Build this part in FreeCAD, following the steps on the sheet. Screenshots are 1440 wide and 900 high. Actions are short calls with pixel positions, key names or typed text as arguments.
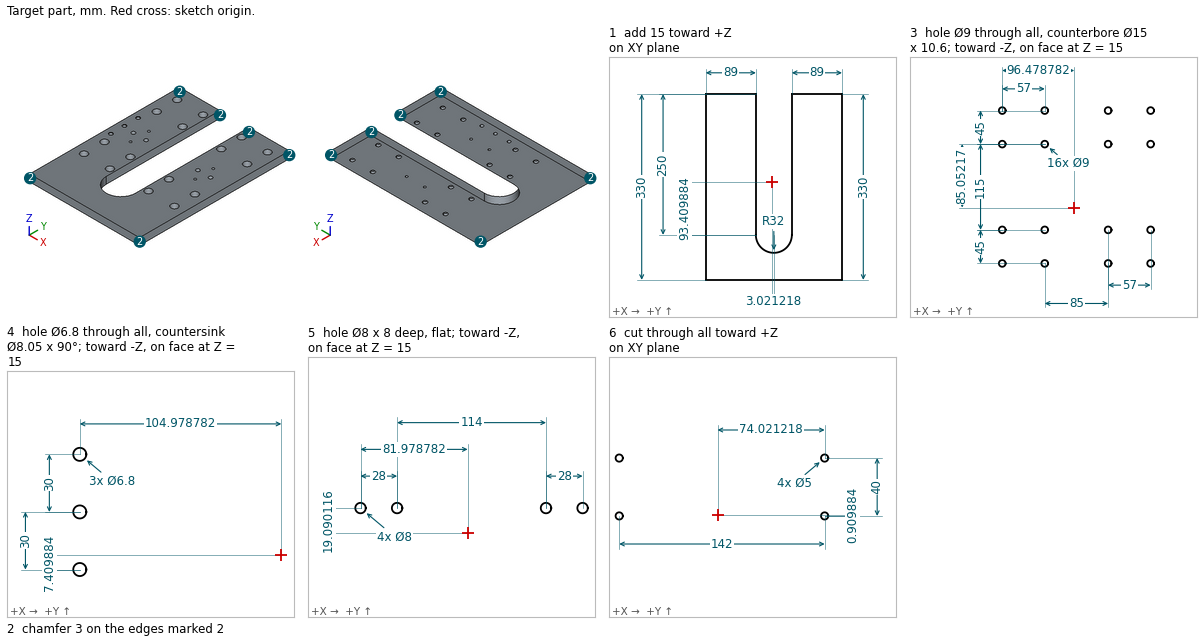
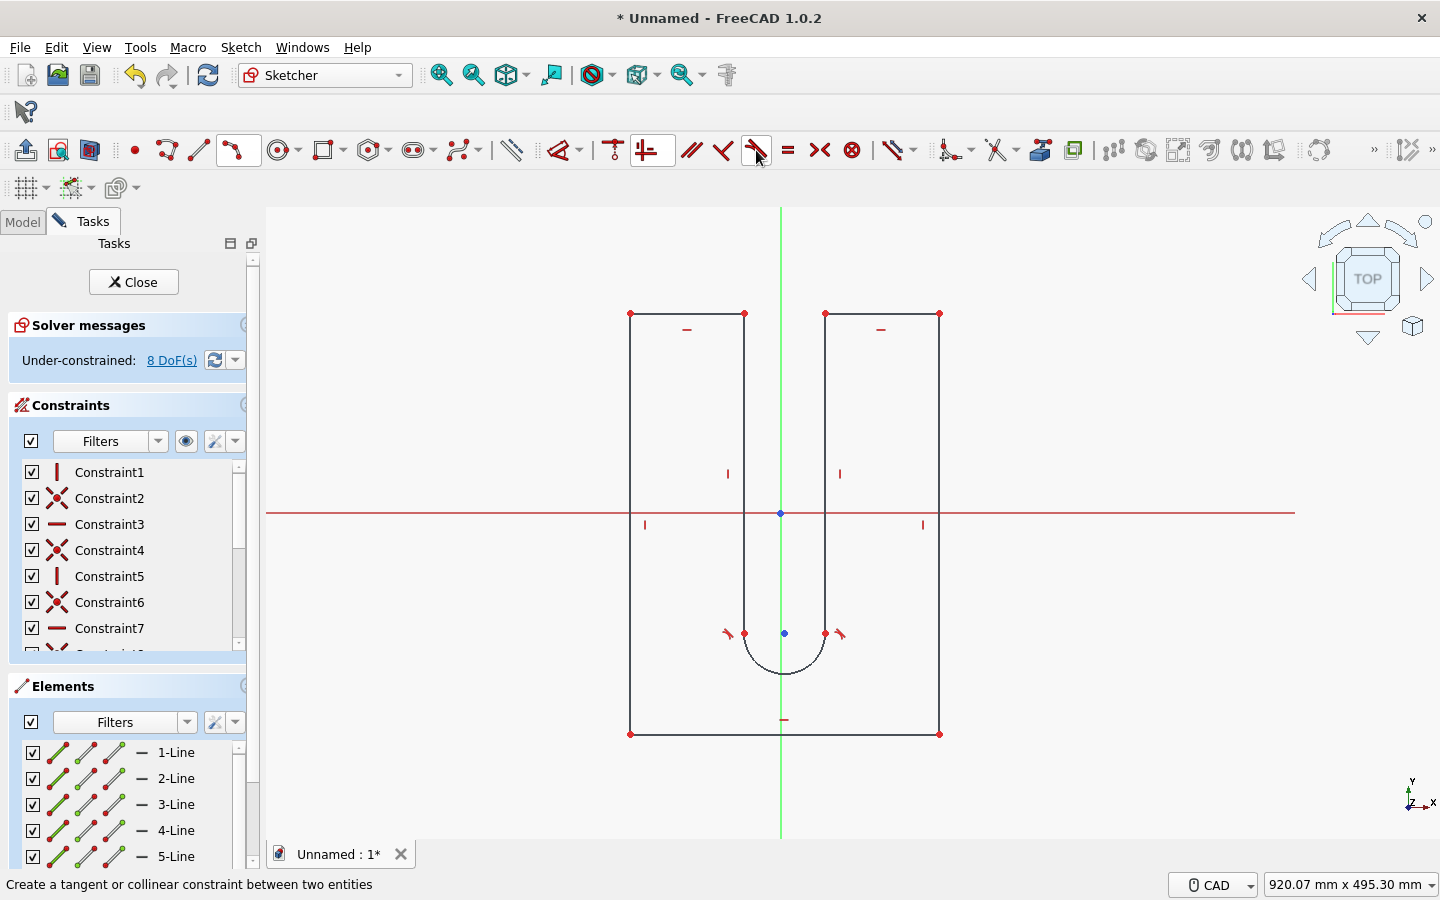
click(558, 150)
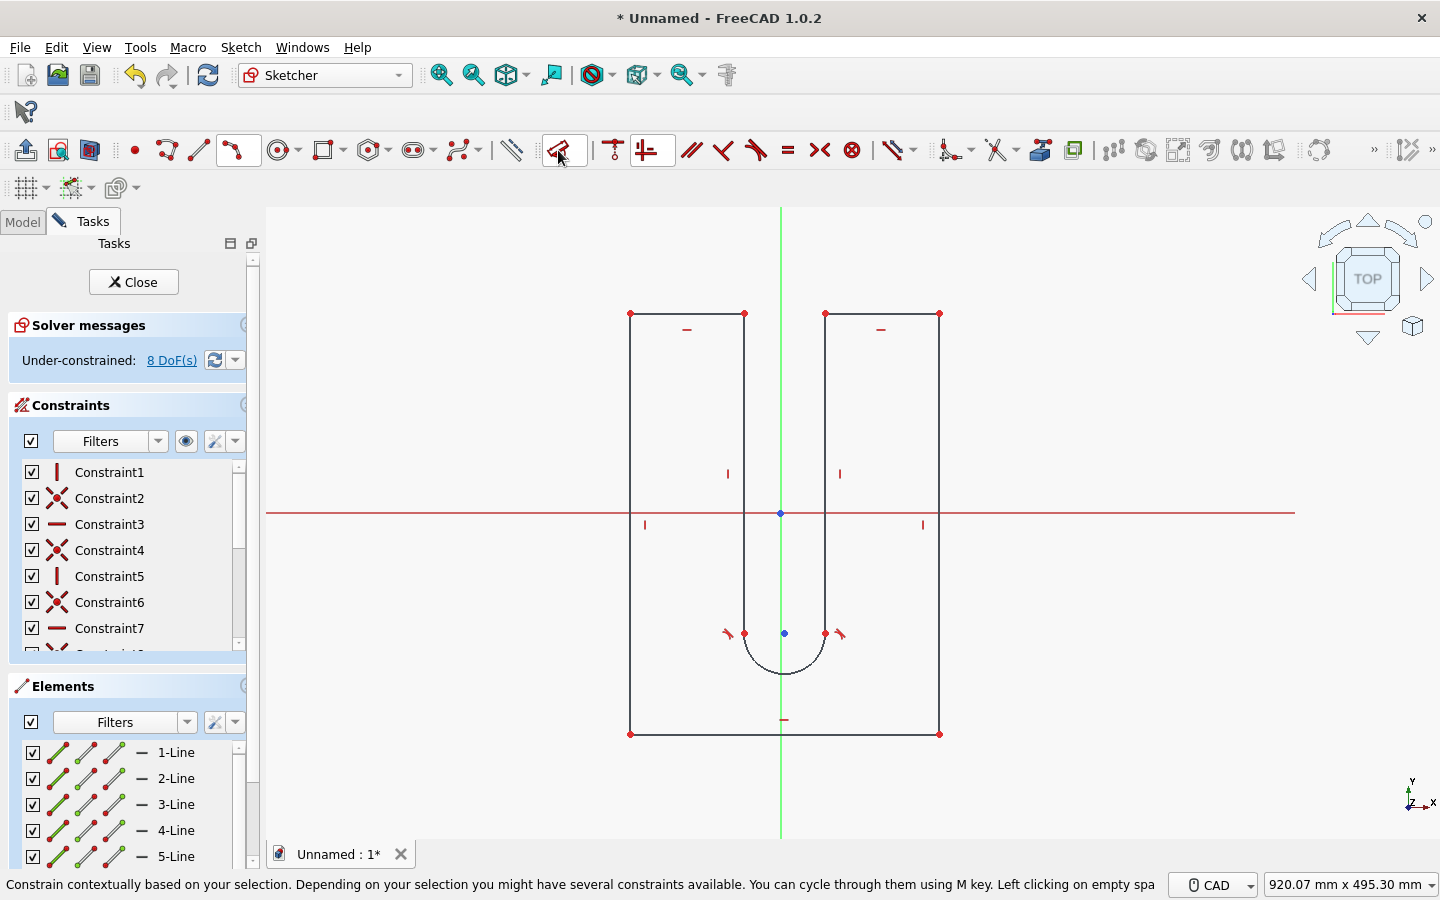
click(761, 666)
click(742, 692)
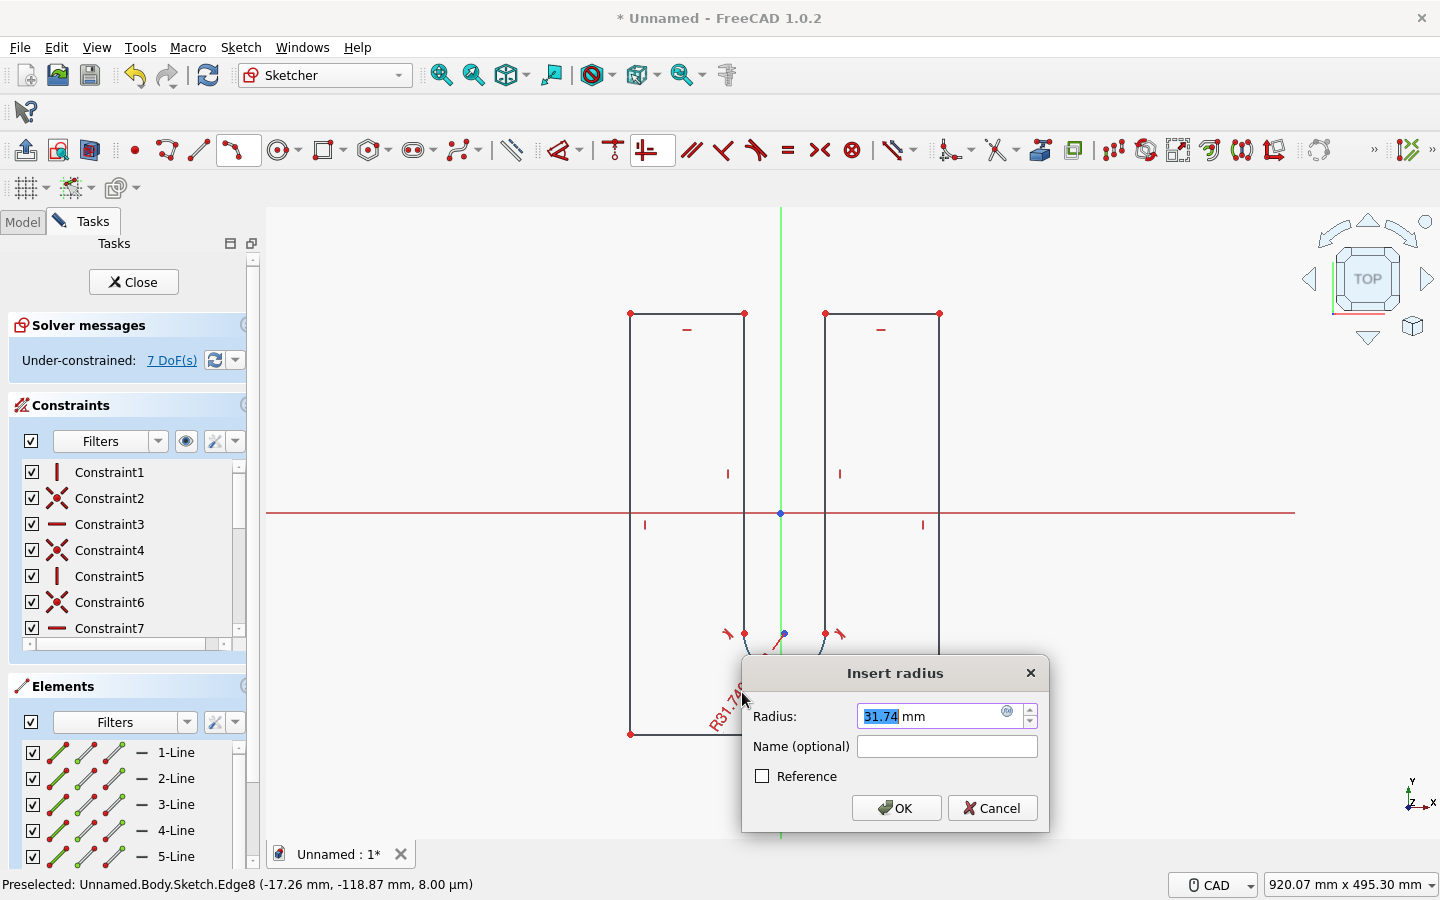
text(32)
key(Return)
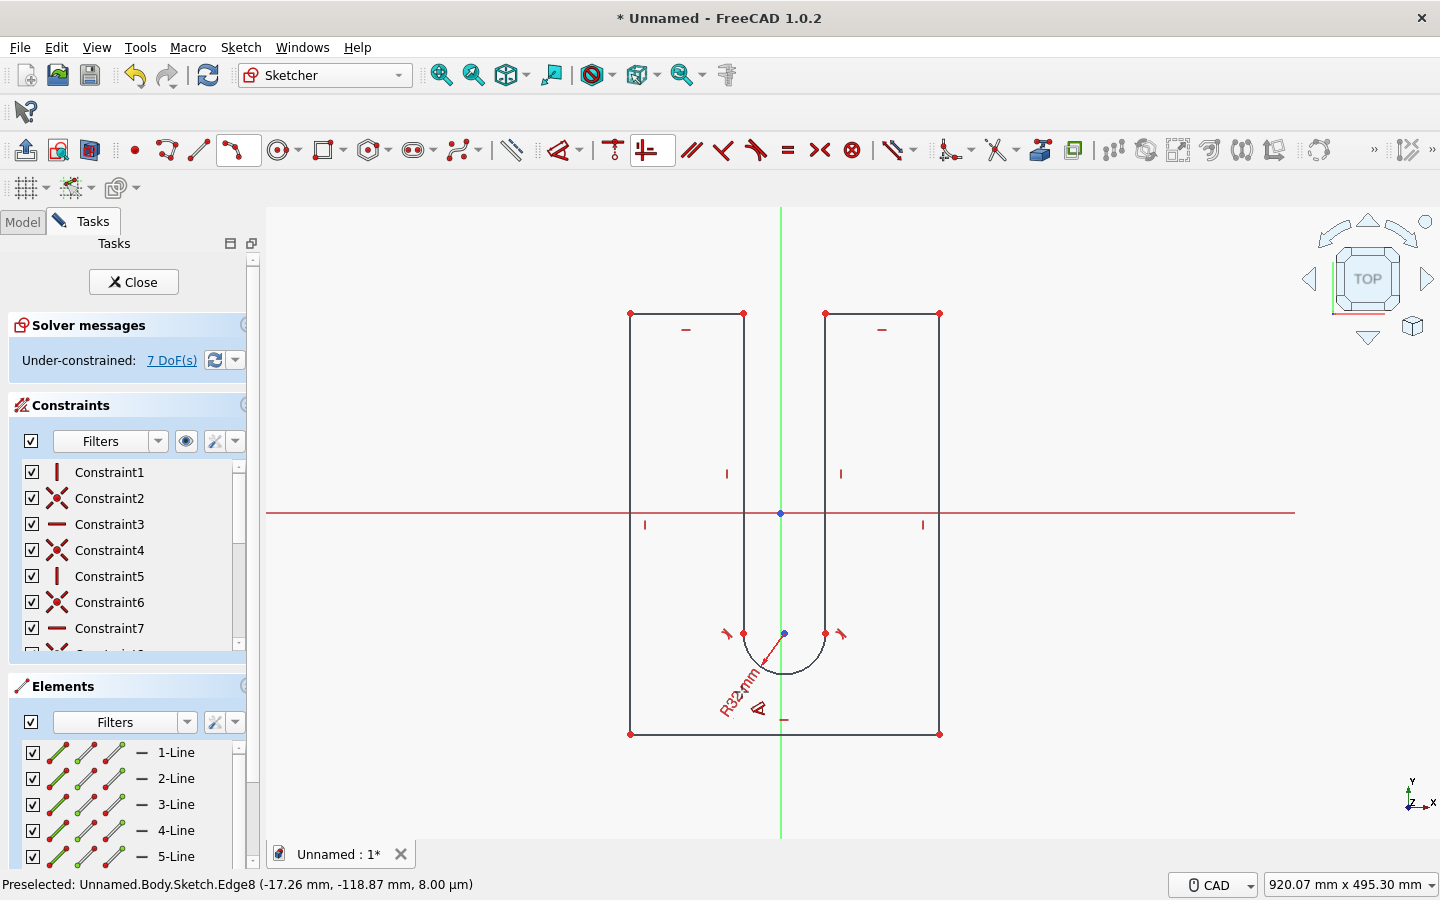
click(710, 314)
click(687, 280)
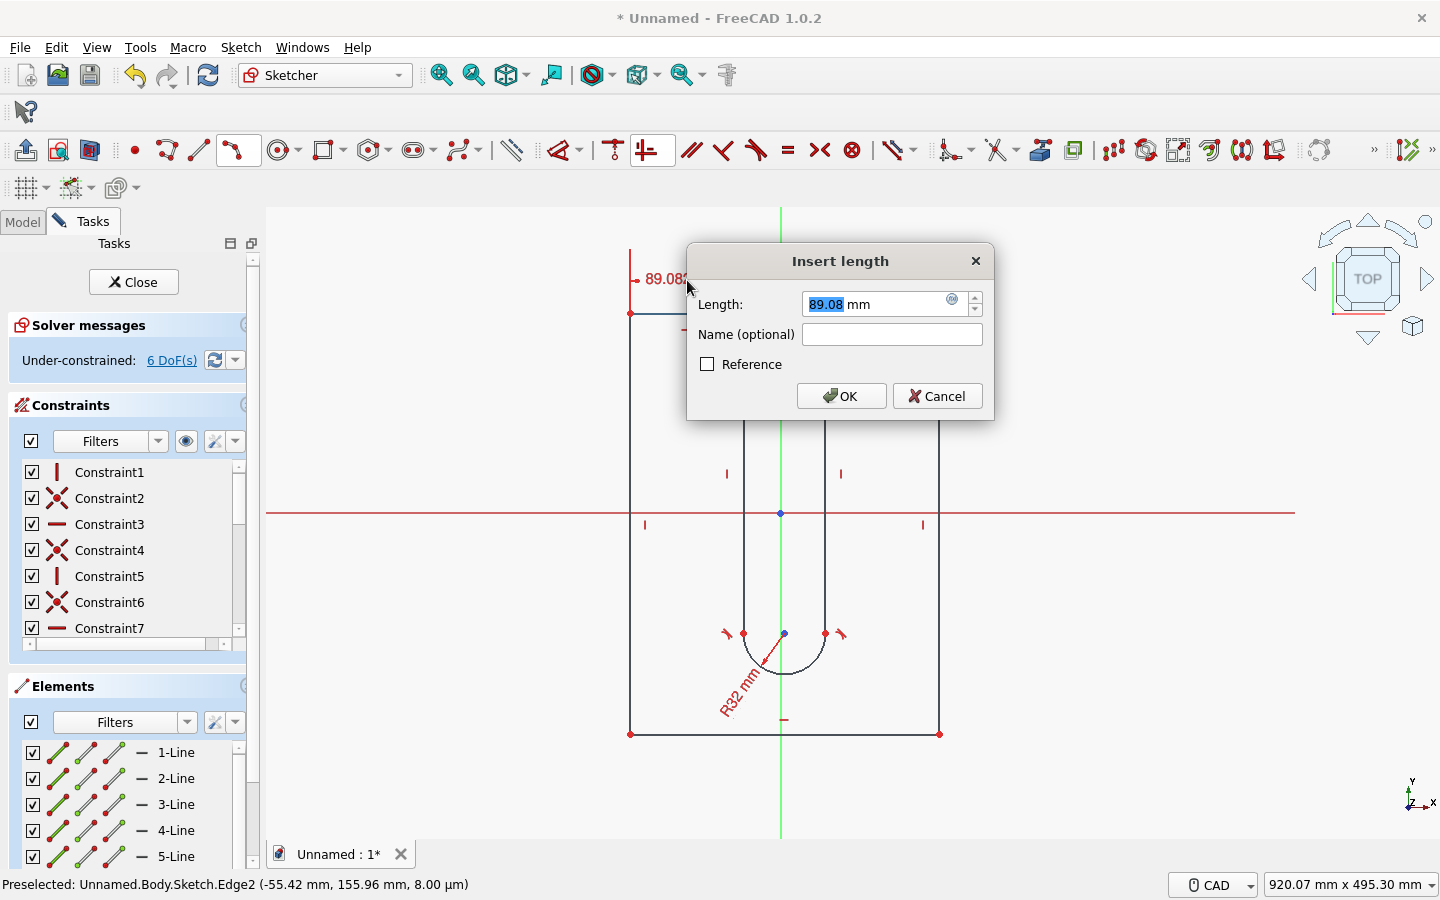
text(89)
key(Return)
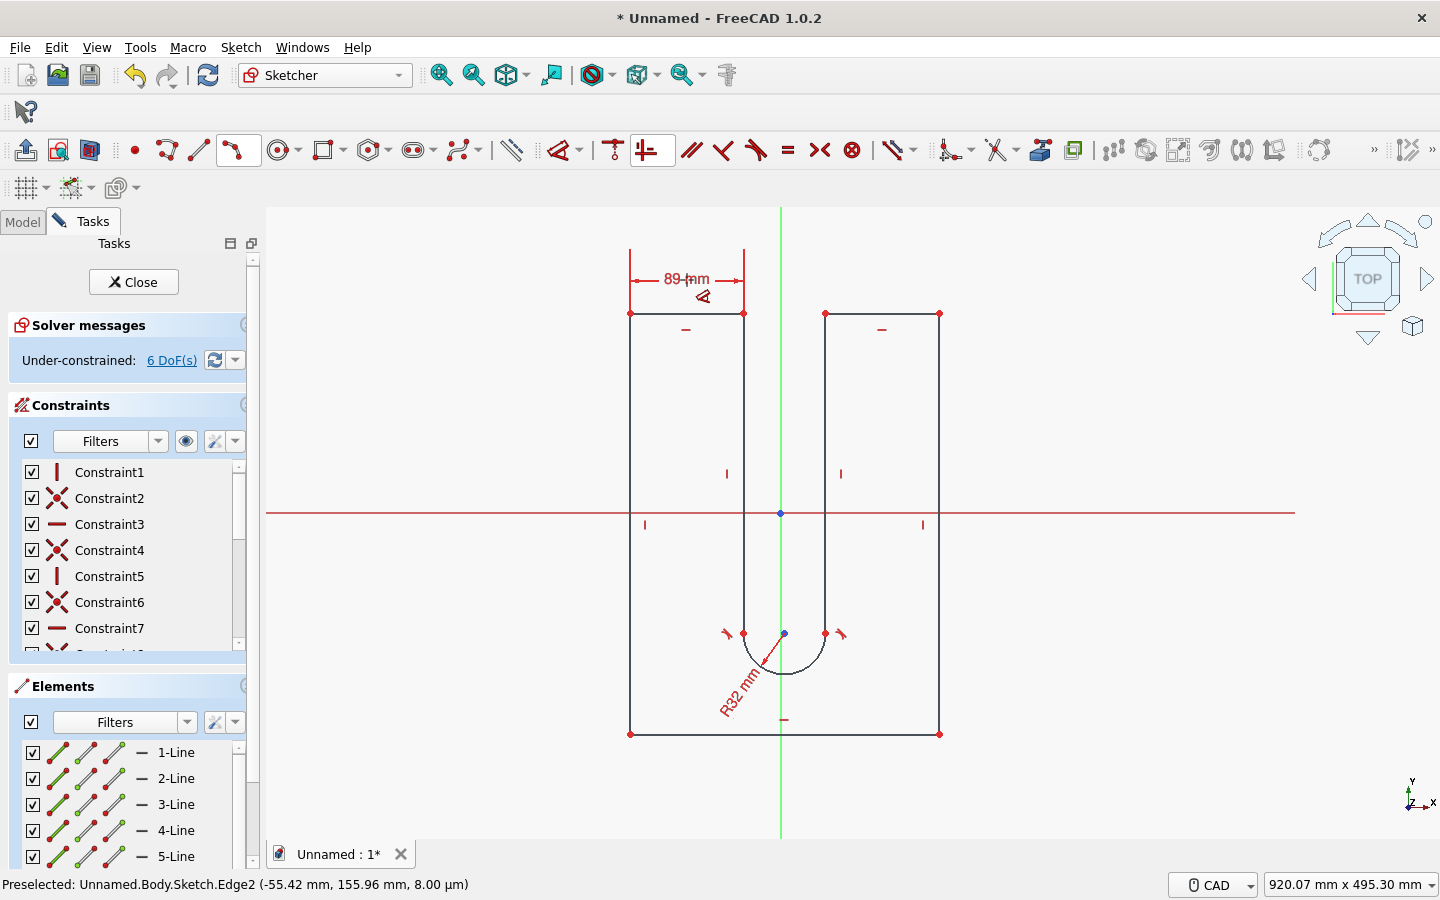
click(905, 314)
click(882, 280)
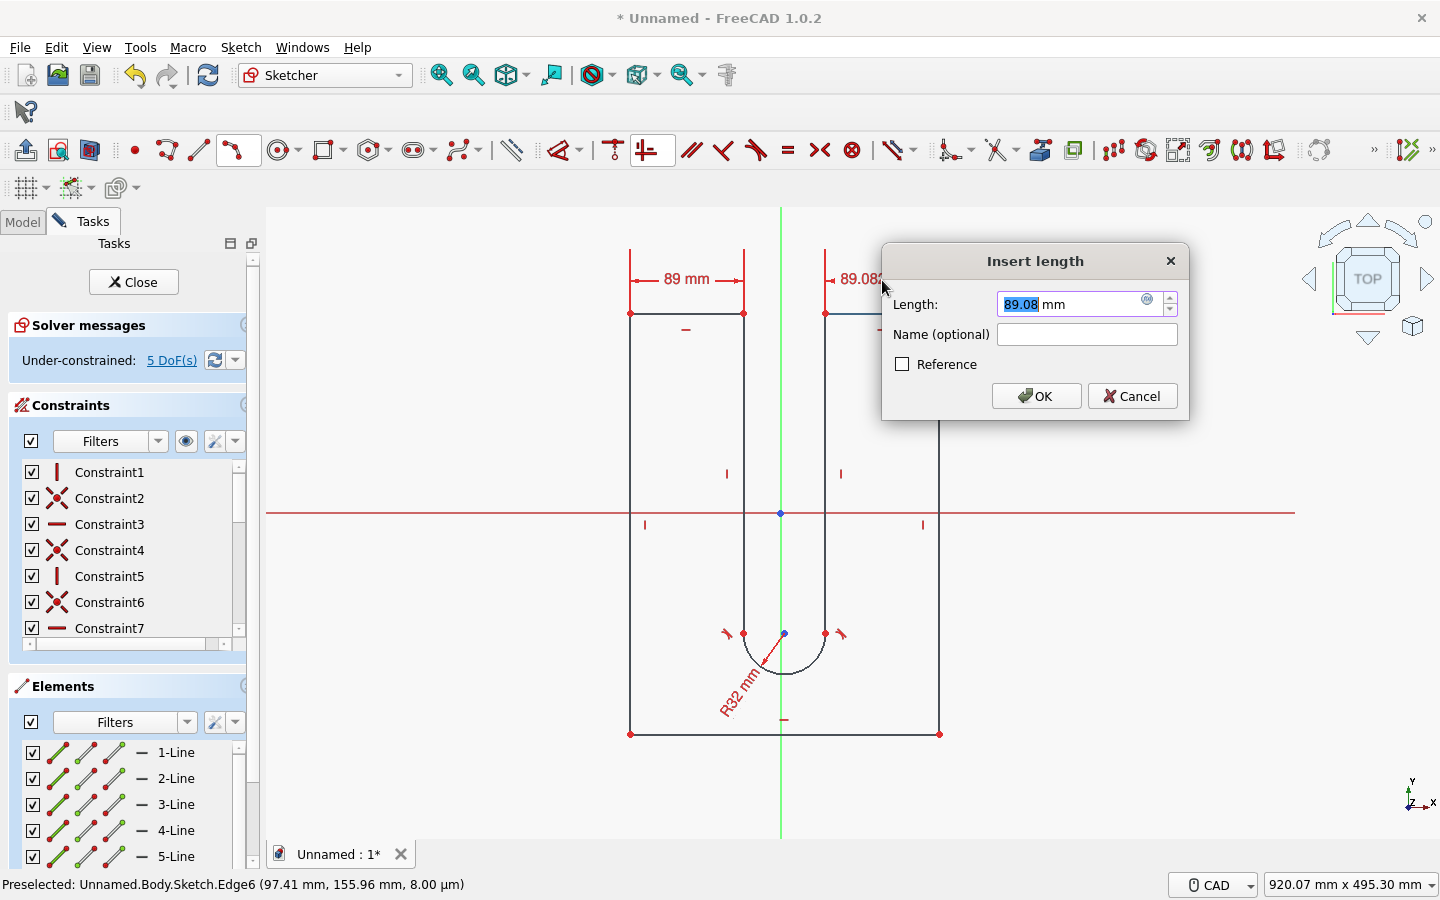
text(89)
key(Return)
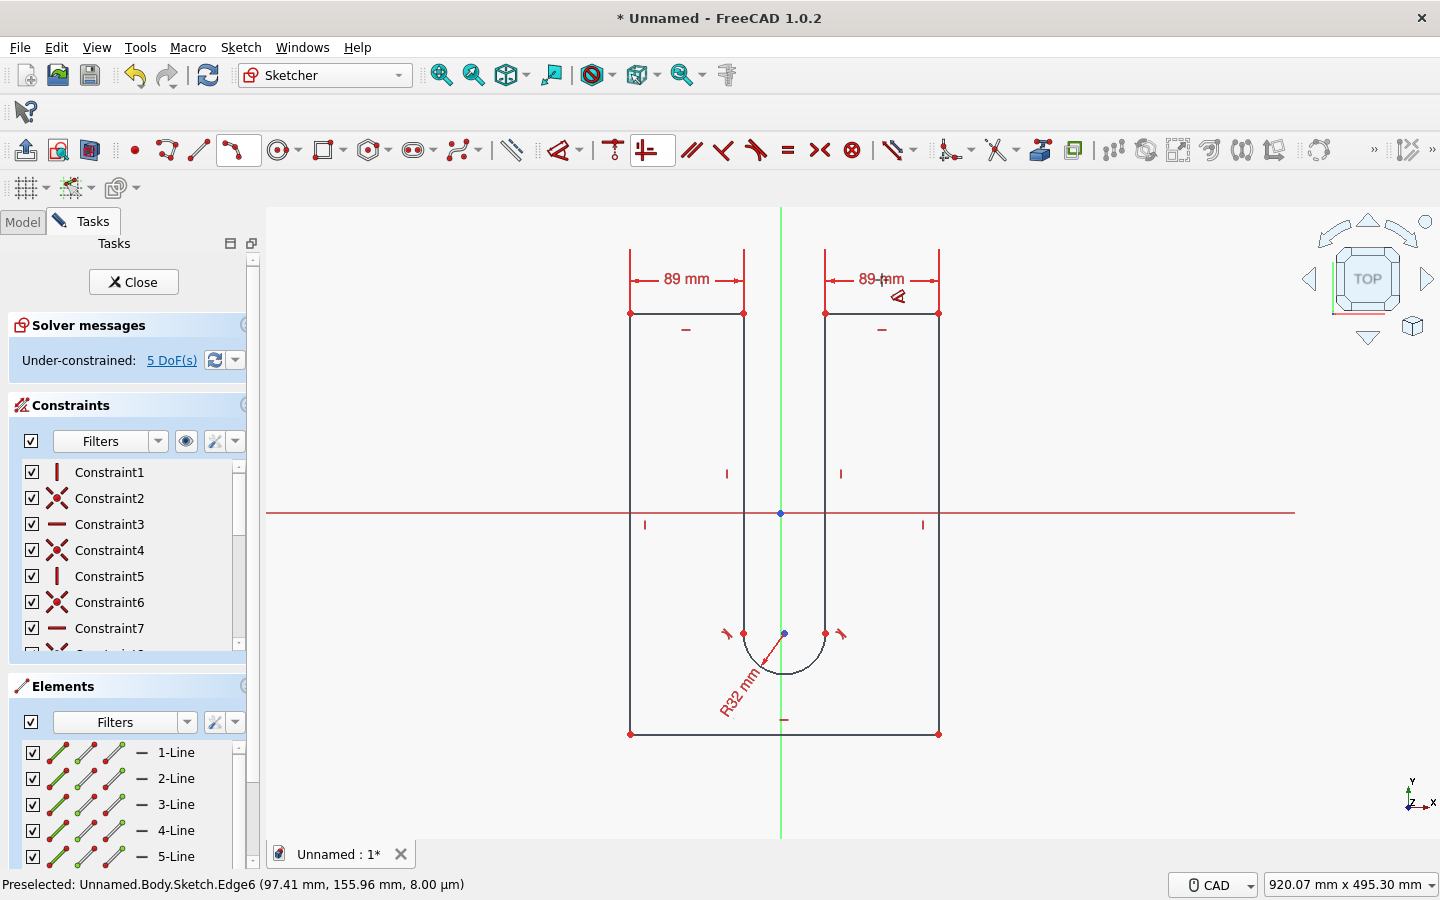
click(744, 538)
click(710, 474)